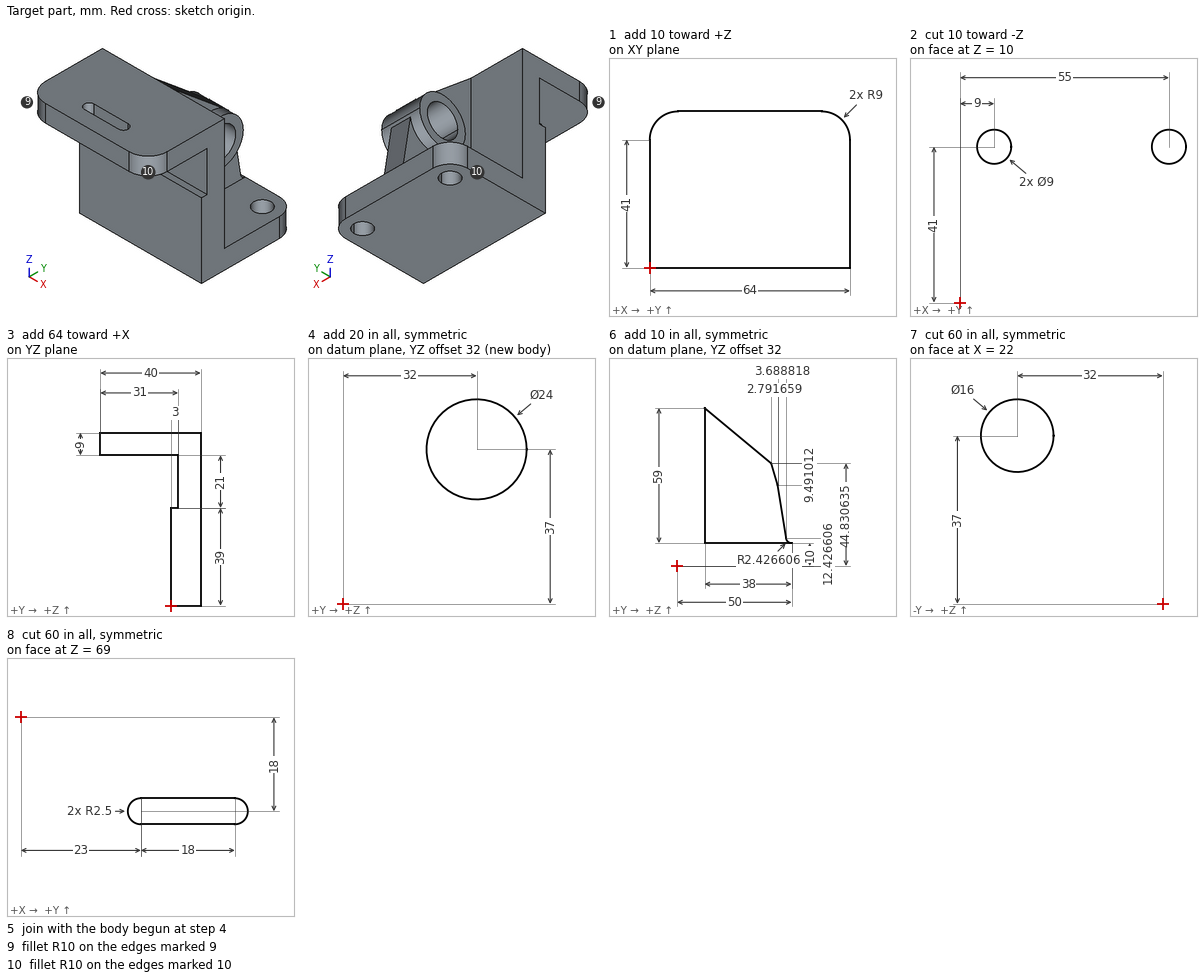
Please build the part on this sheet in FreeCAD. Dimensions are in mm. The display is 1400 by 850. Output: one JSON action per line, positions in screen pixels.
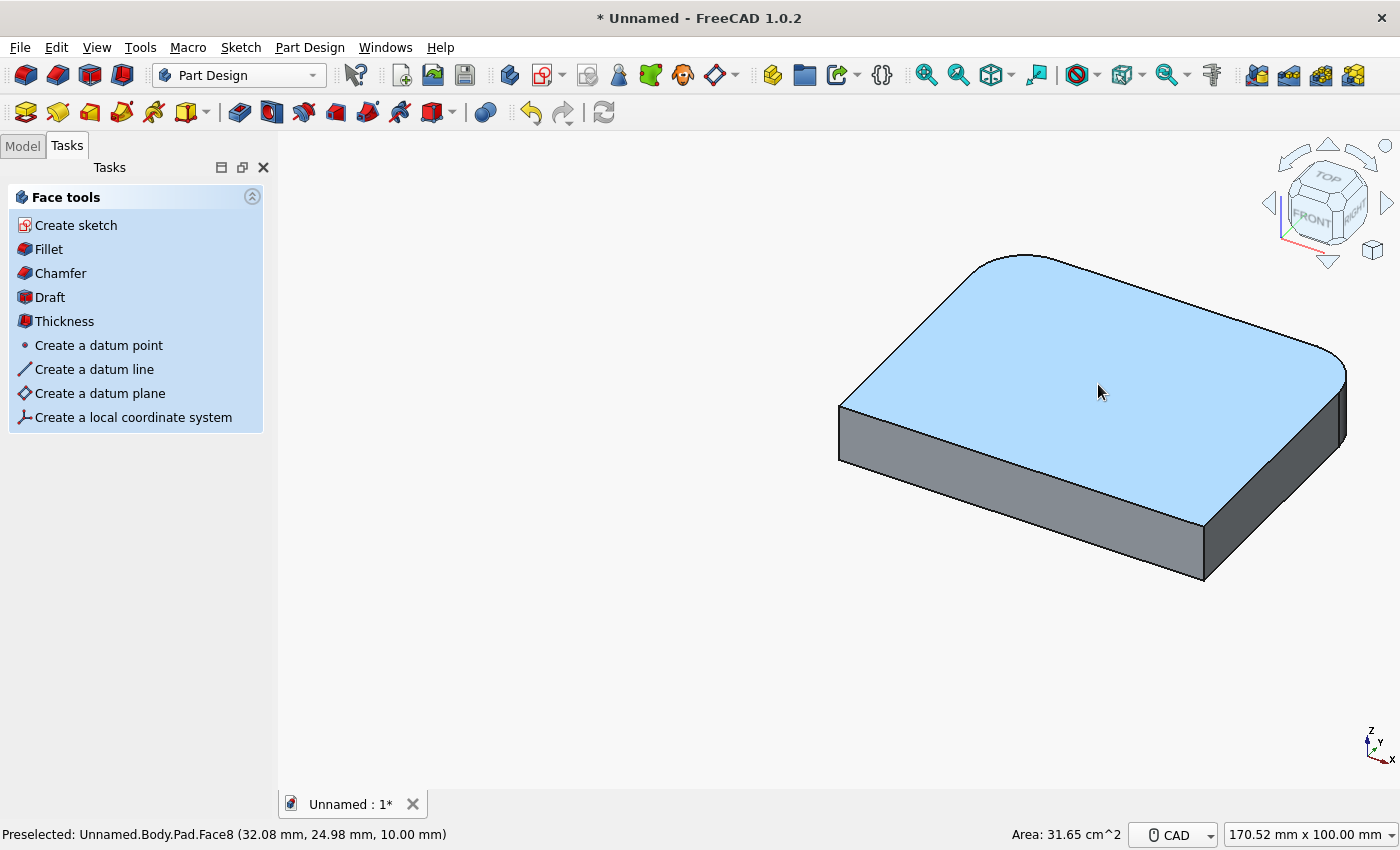
{"action": "left_click", "coordinate": [542, 76]}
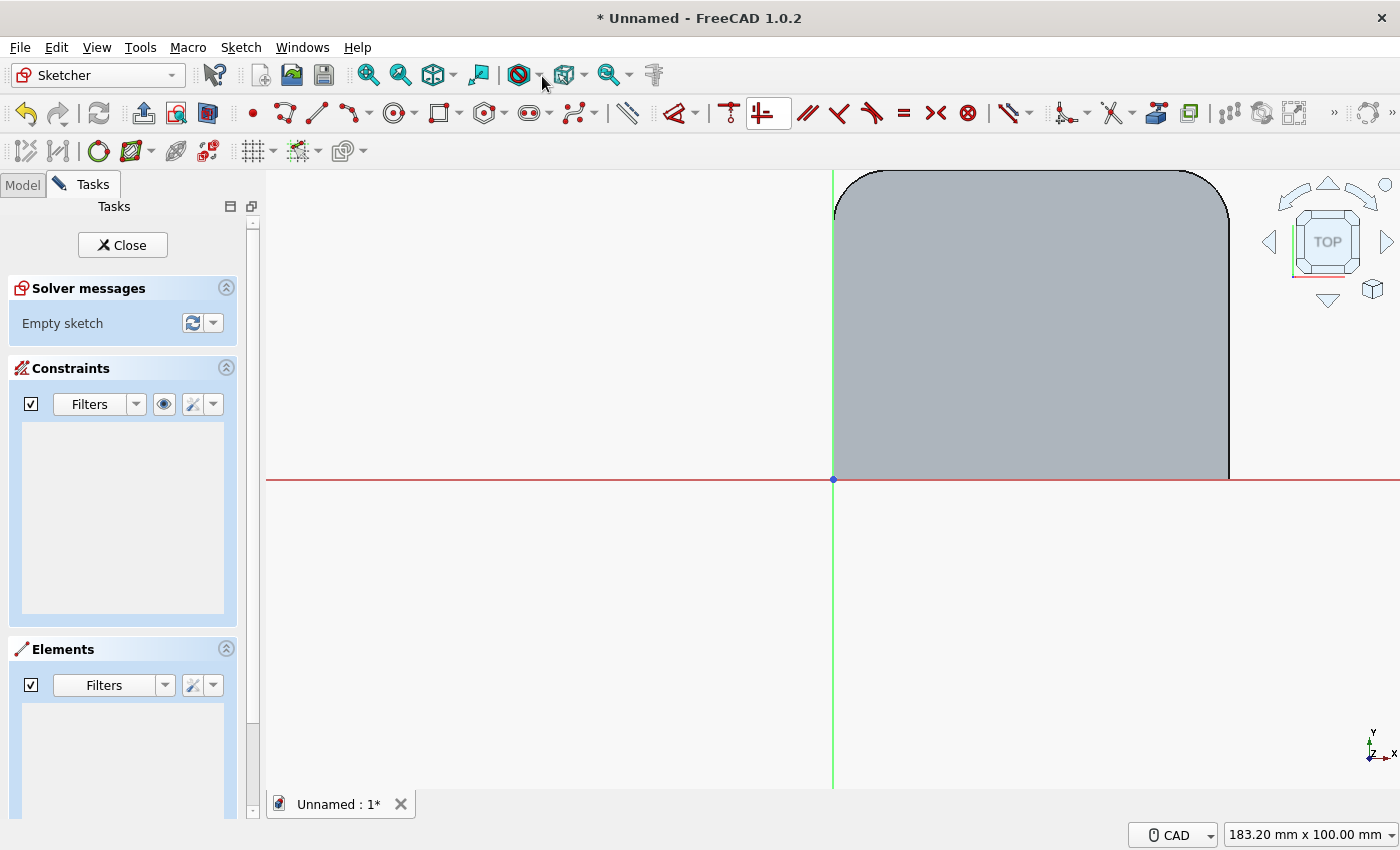
{"action": "scroll", "coordinate": [294, 761], "scroll_direction": "down", "scroll_amount": 1}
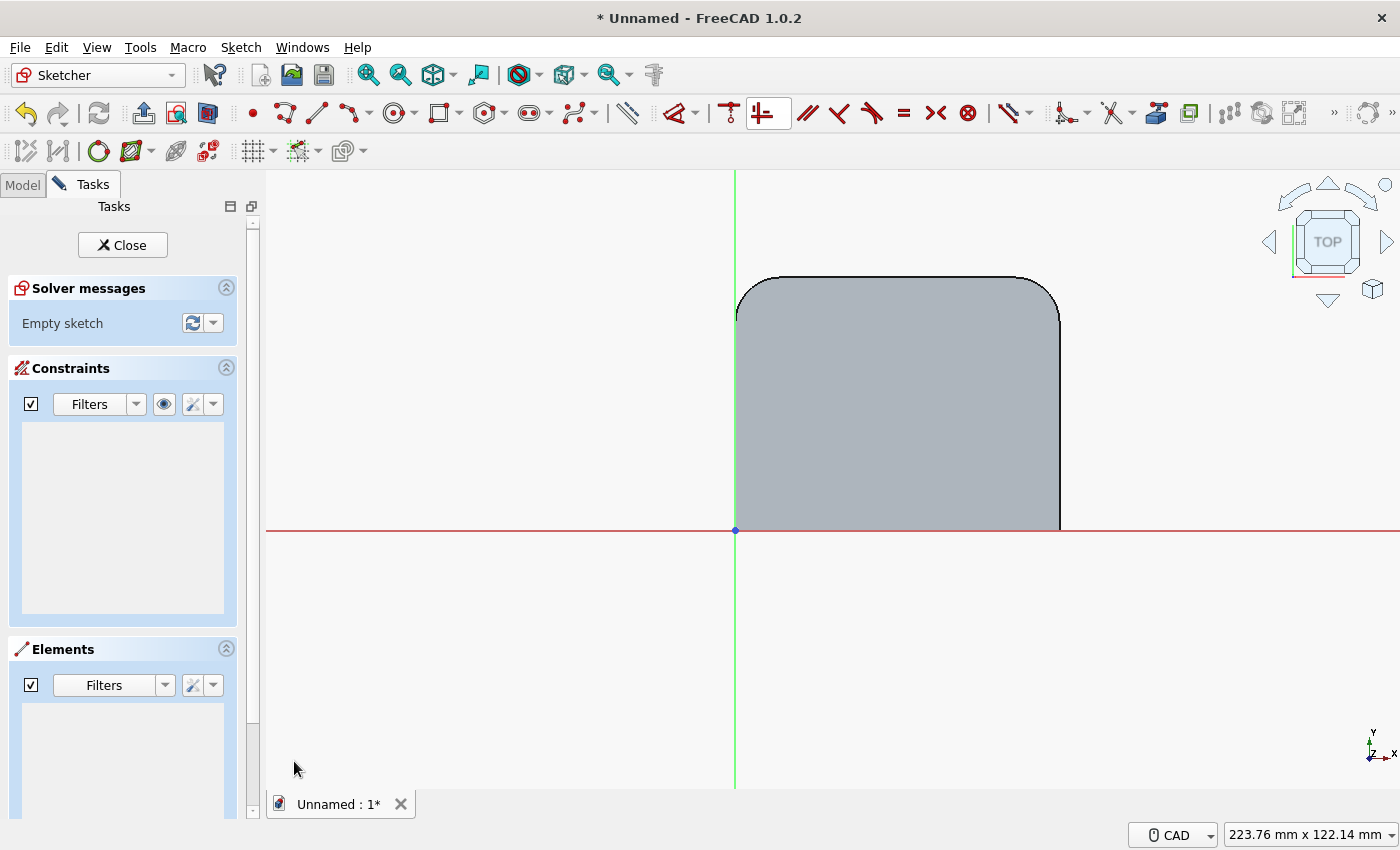
{"action": "scroll", "coordinate": [1034, 337], "scroll_direction": "up", "scroll_amount": 3}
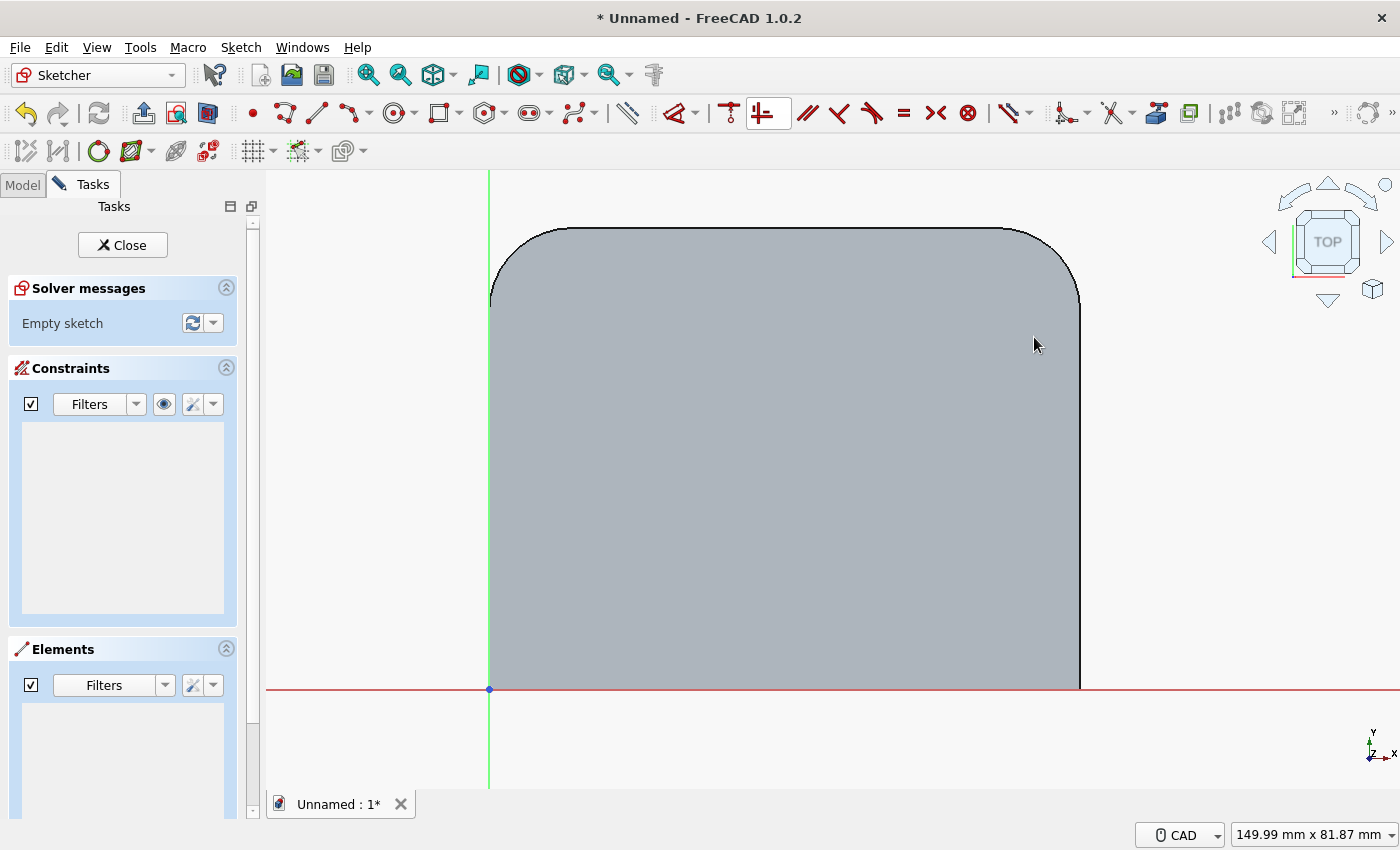
{"action": "left_click", "coordinate": [394, 114]}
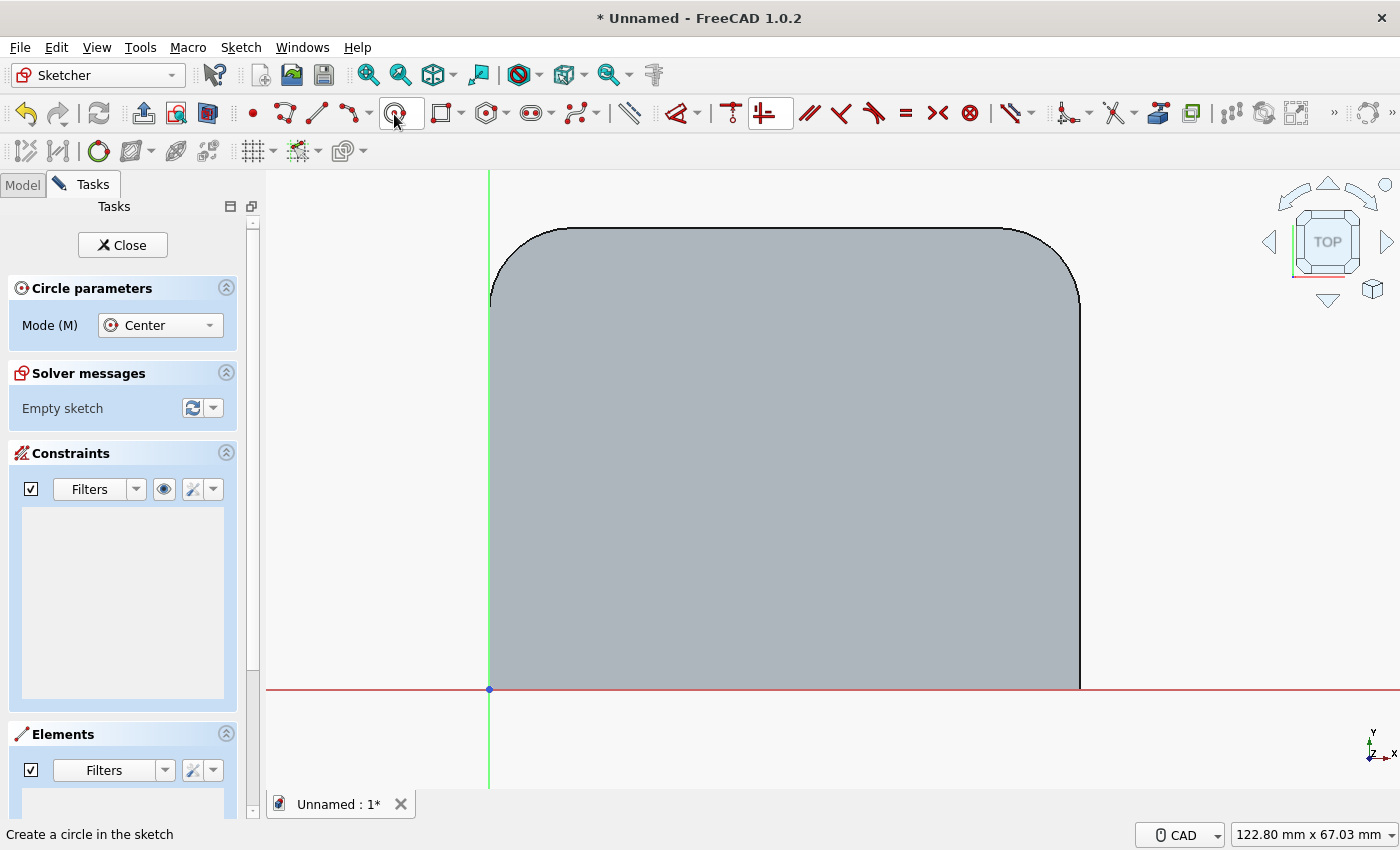
{"action": "left_click", "coordinate": [572, 311]}
{"action": "mouse_move", "coordinate": [602, 282]}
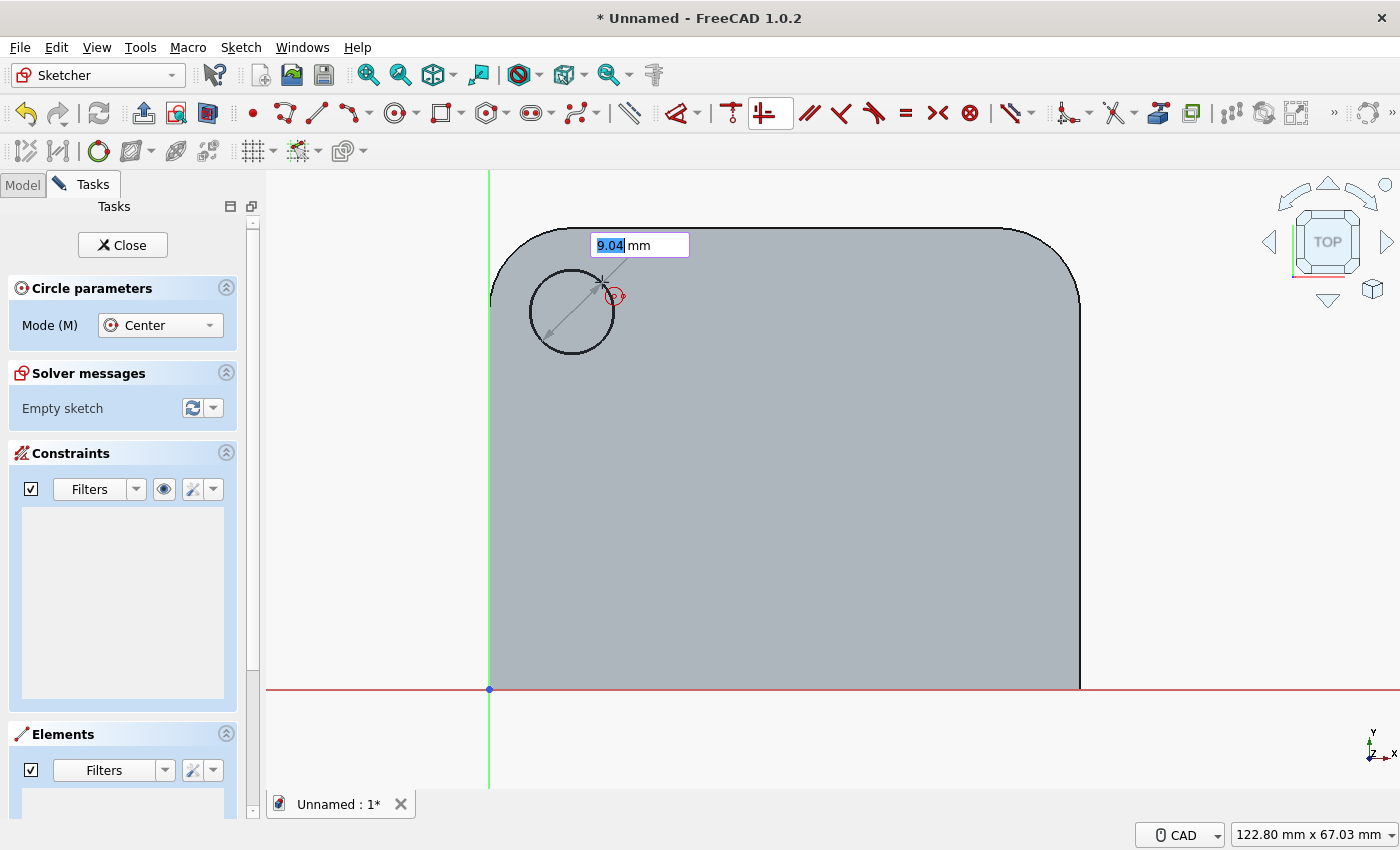
{"action": "type", "text": "9"}
{"action": "key", "text": "Return"}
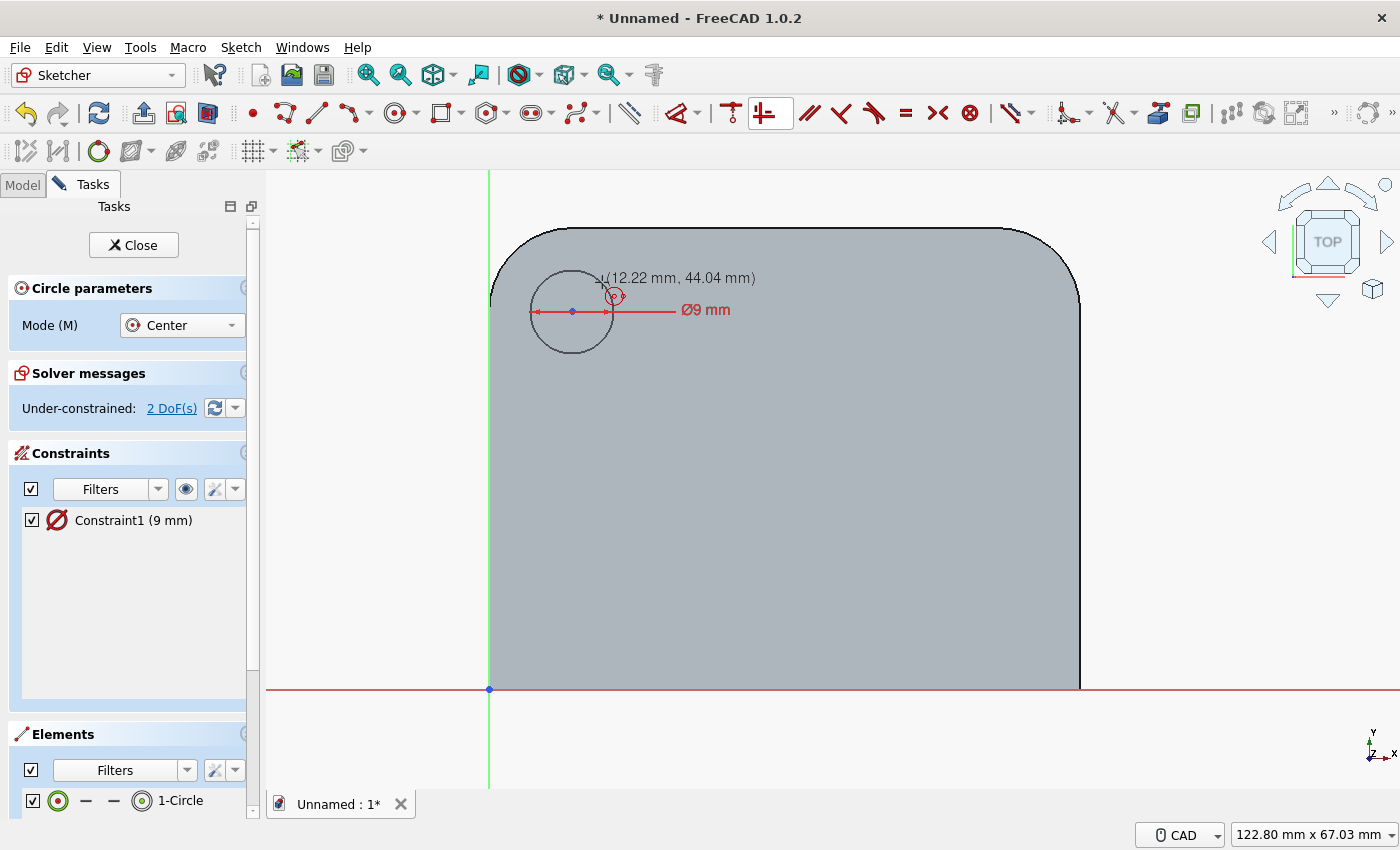
{"action": "left_click", "coordinate": [997, 311]}
{"action": "mouse_move", "coordinate": [1026, 282]}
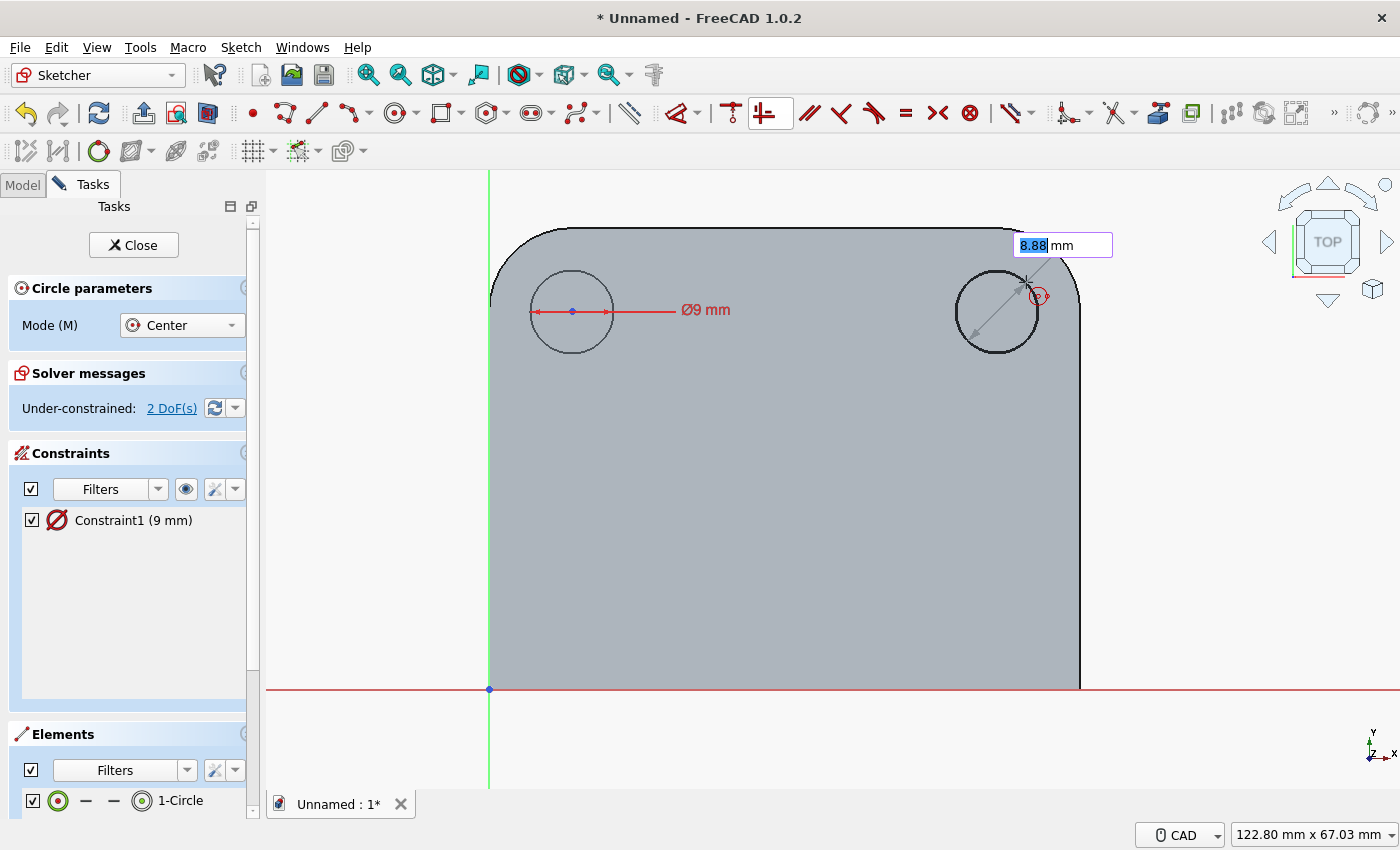
{"action": "type", "text": "9"}
{"action": "key", "text": "Return"}
{"action": "key", "text": "Escape"}